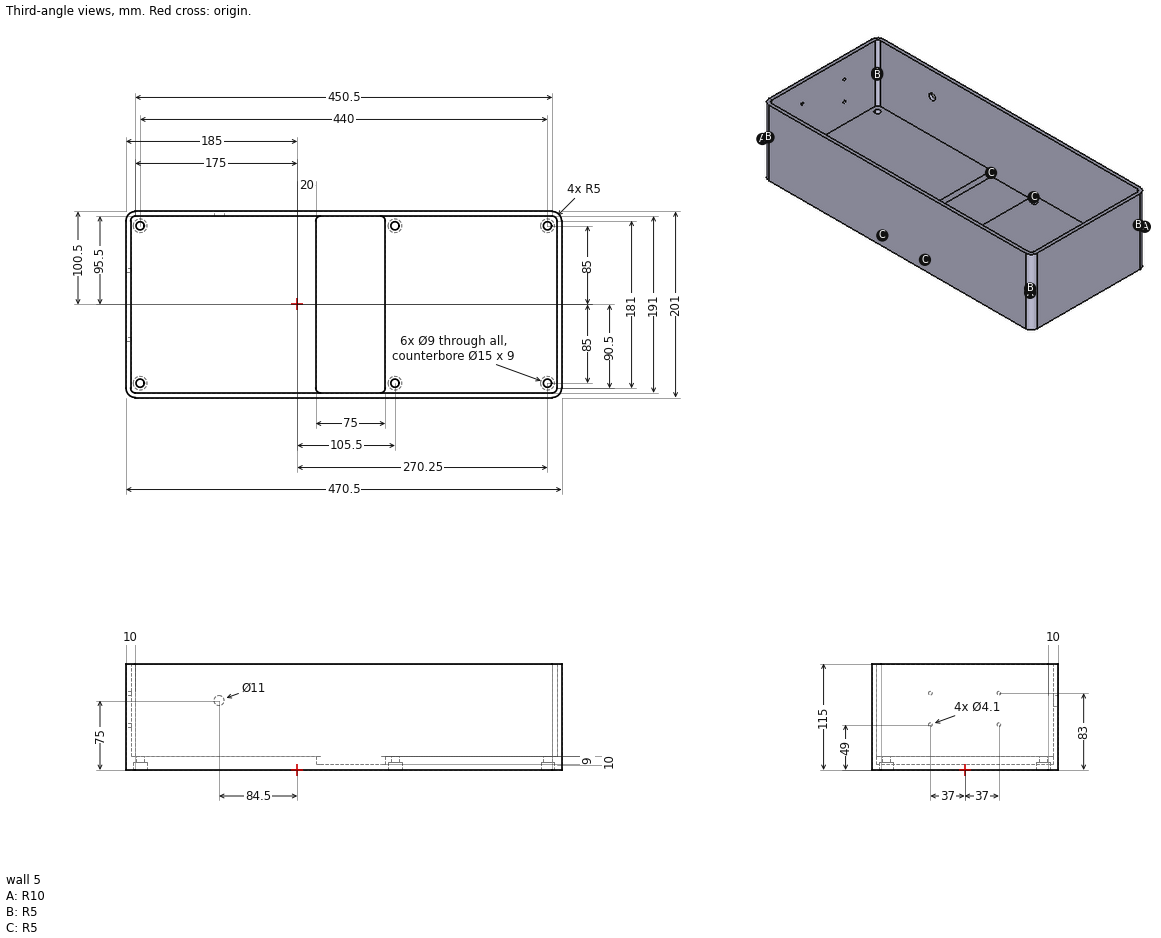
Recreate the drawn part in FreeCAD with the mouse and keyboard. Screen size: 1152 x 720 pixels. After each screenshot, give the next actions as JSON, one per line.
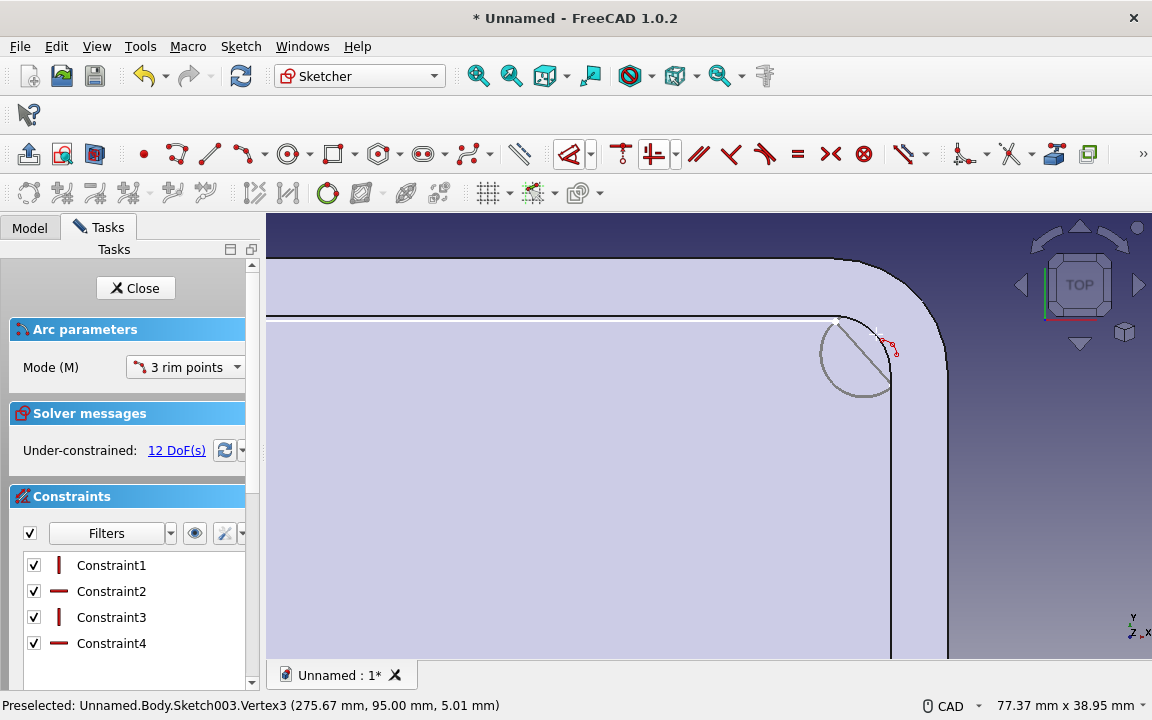
{"action": "left_click", "coordinate": [874, 332]}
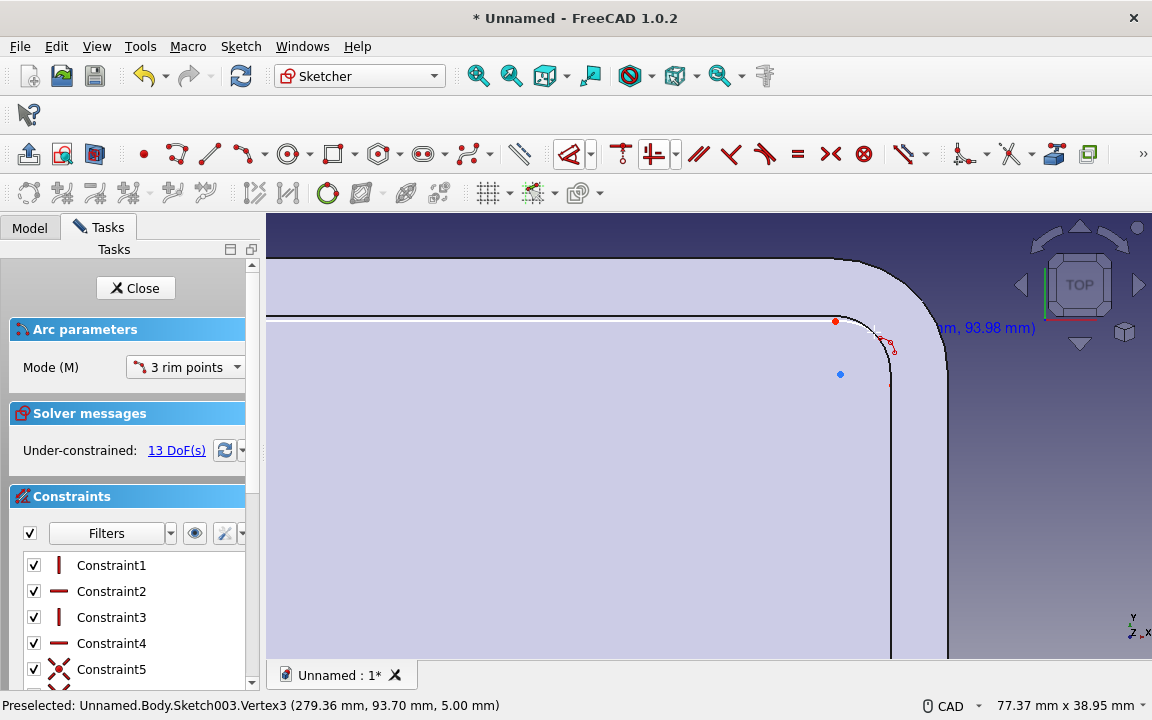
{"action": "scroll", "coordinate": [879, 339], "scroll_direction": "down", "scroll_amount": 12}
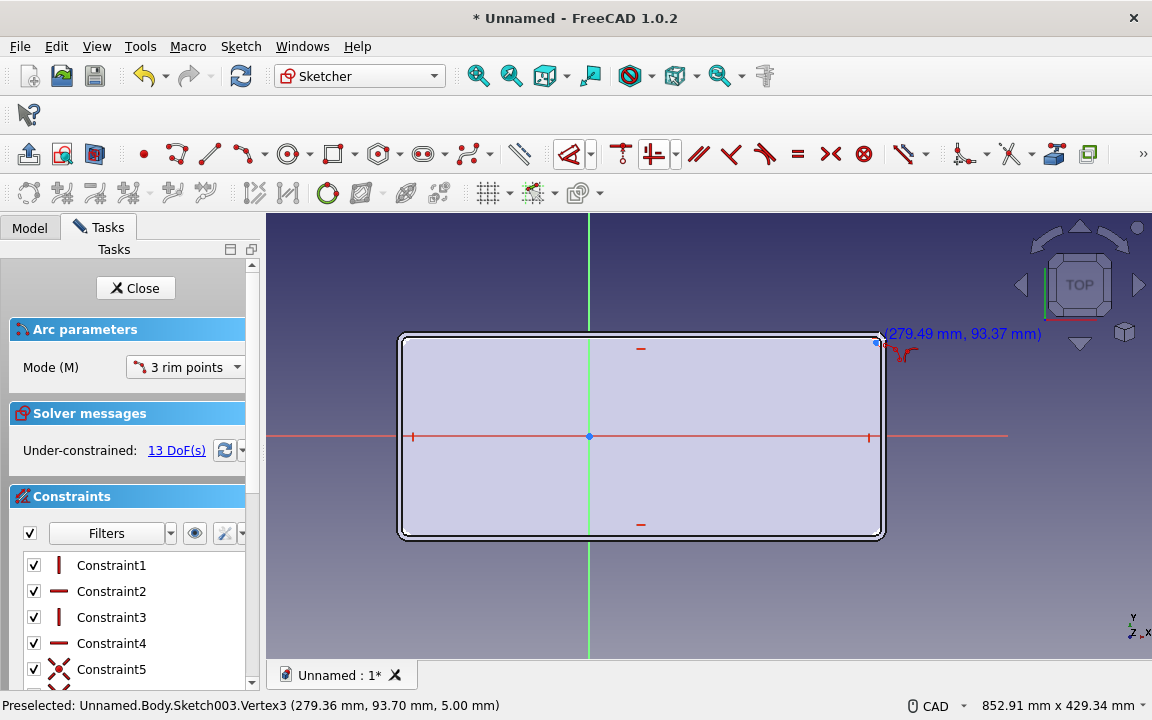
{"action": "scroll", "coordinate": [408, 337], "scroll_direction": "up", "scroll_amount": 4}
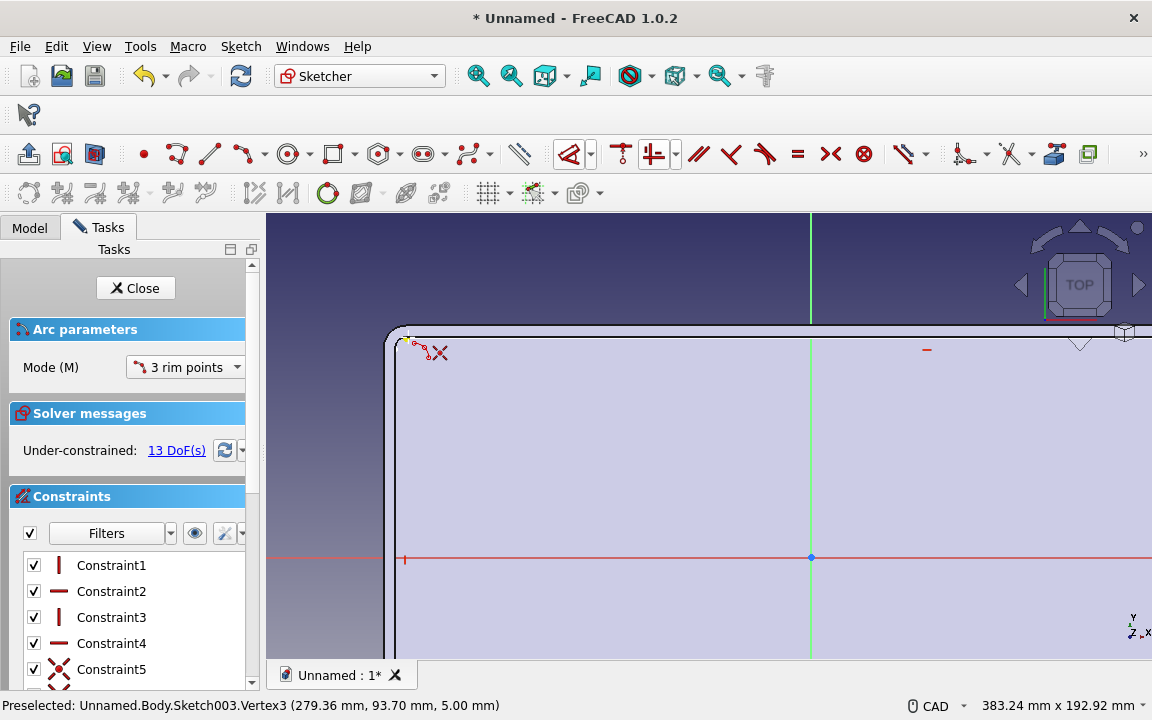
{"action": "left_click", "coordinate": [407, 338]}
{"action": "left_click", "coordinate": [395, 349]}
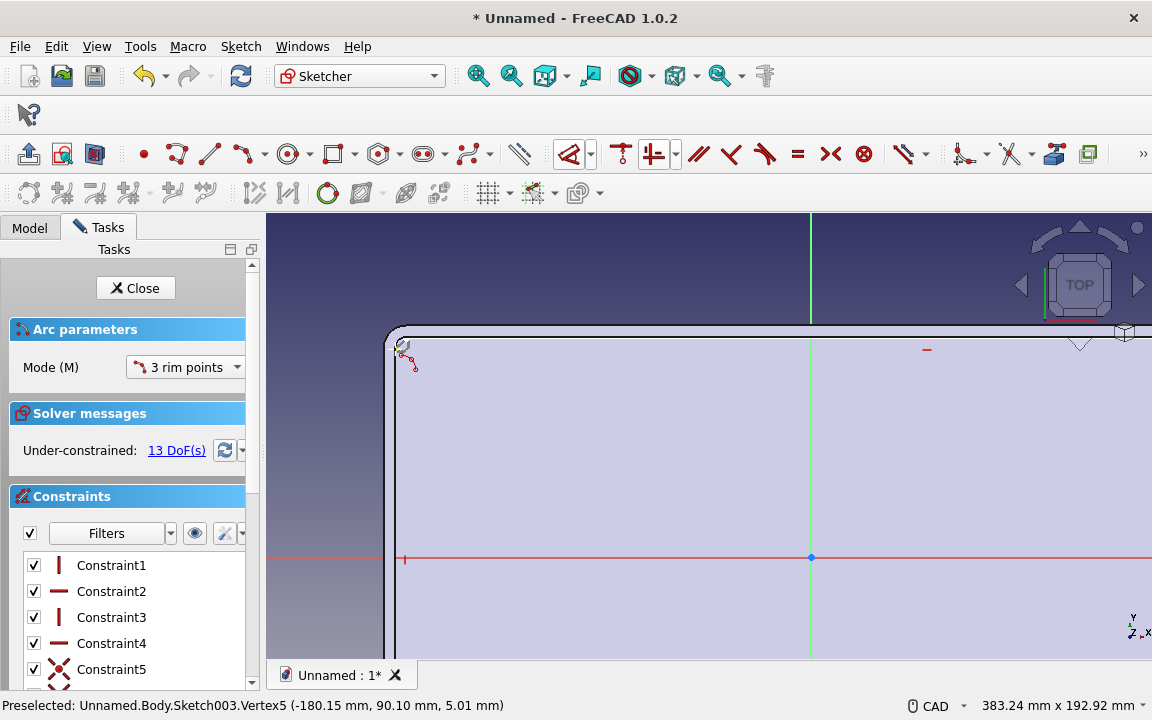
{"action": "scroll", "coordinate": [399, 340], "scroll_direction": "up", "scroll_amount": 8}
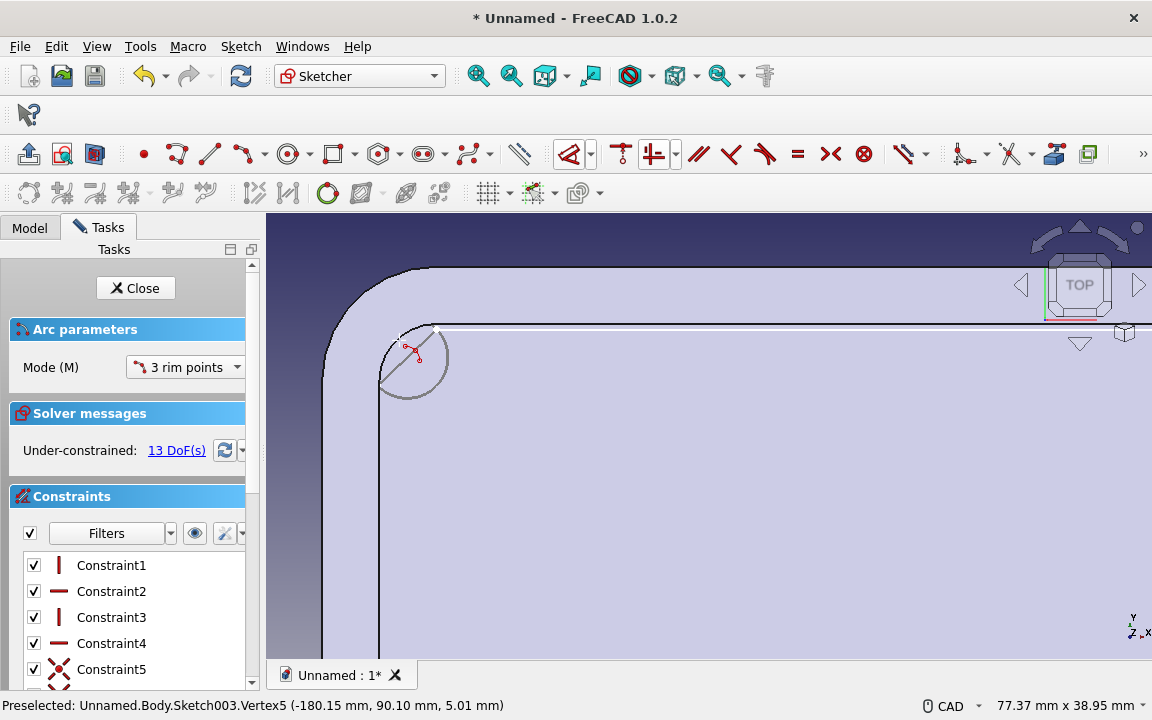
{"action": "left_click", "coordinate": [396, 341]}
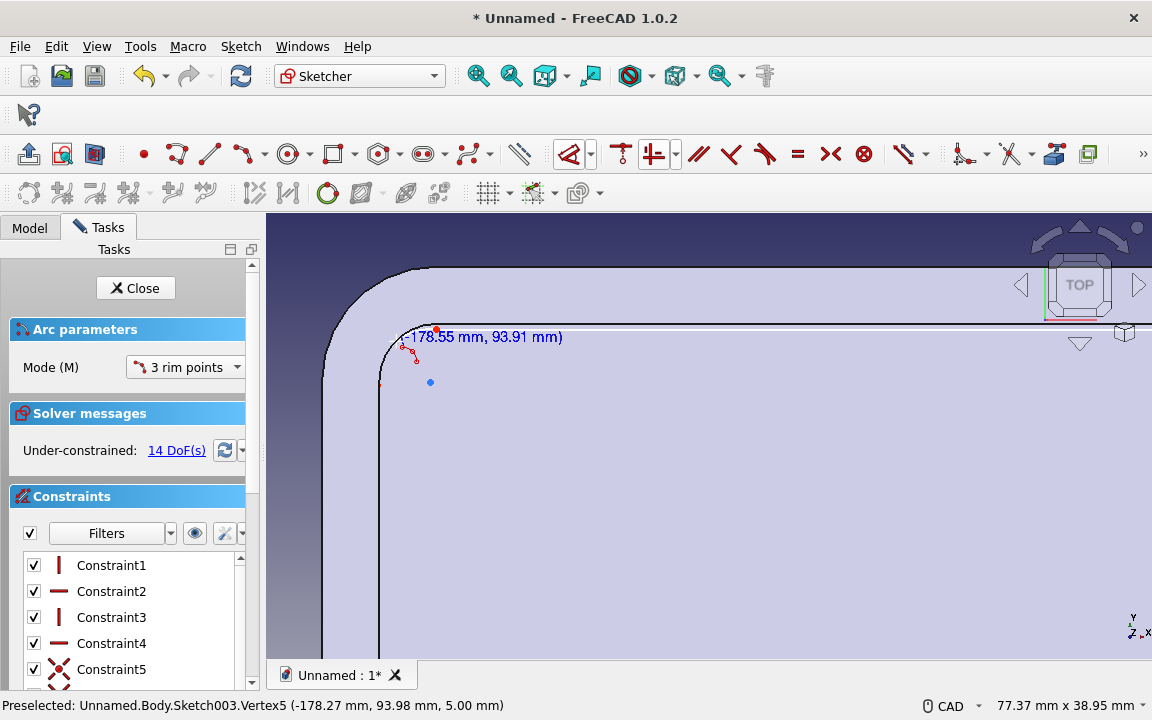
{"action": "scroll", "coordinate": [404, 338], "scroll_direction": "down", "scroll_amount": 12}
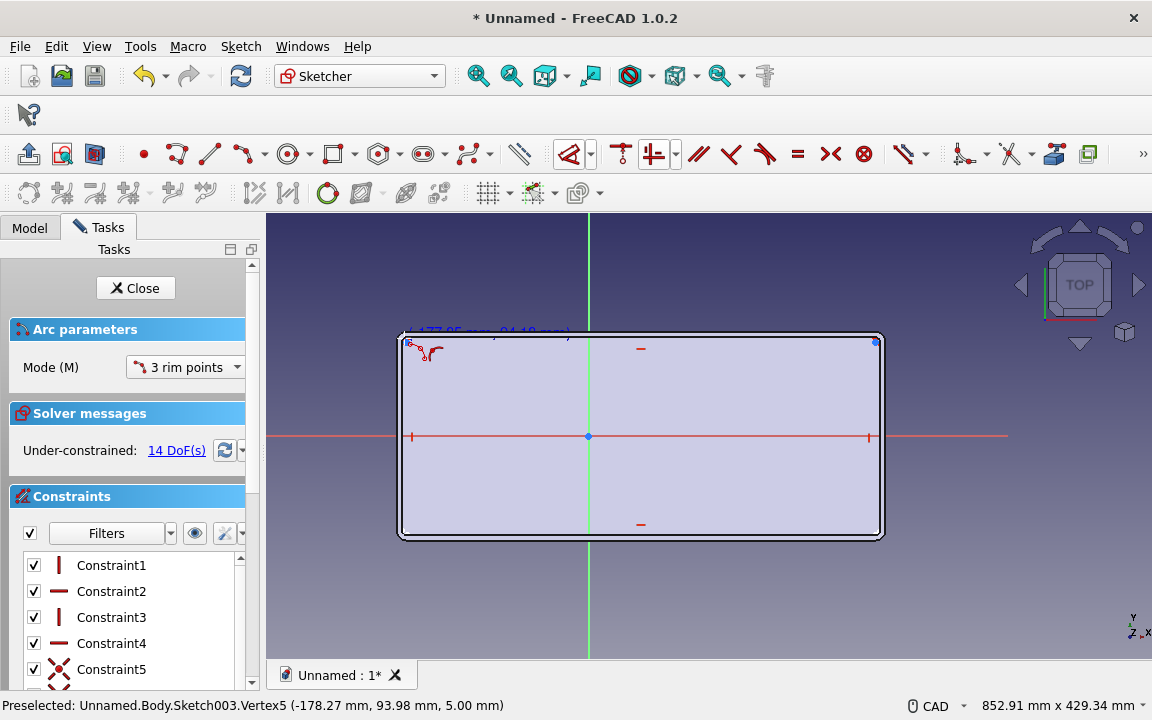
{"action": "scroll", "coordinate": [402, 530], "scroll_direction": "up", "scroll_amount": 4}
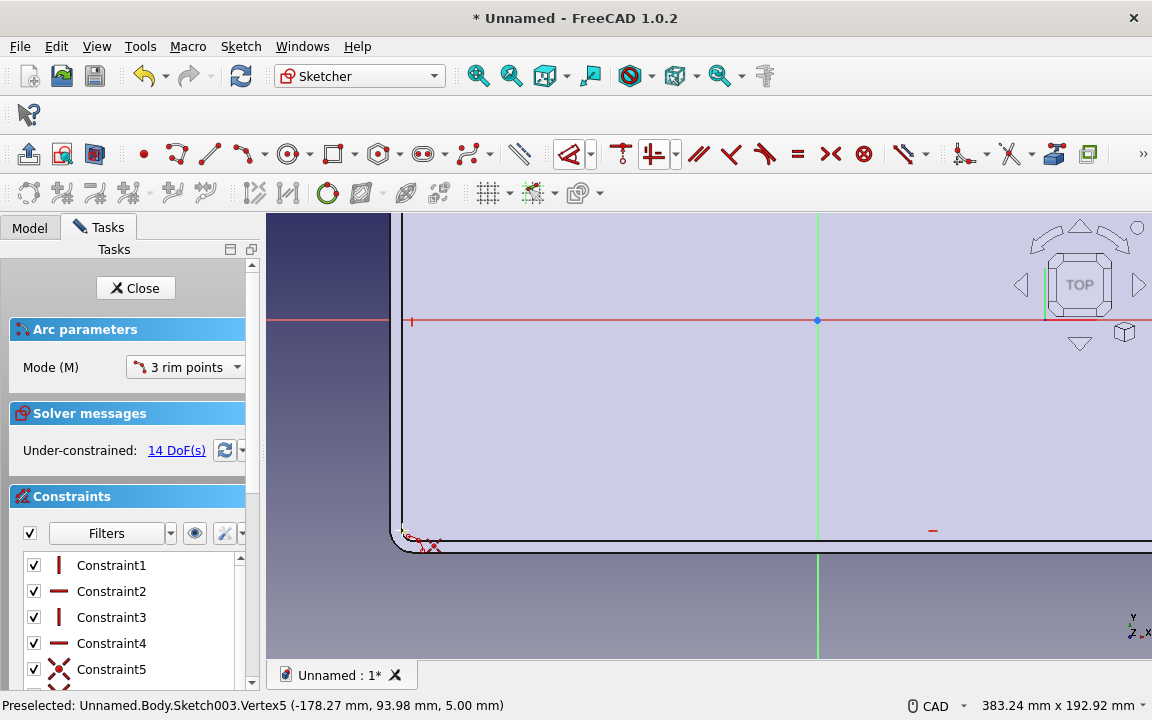
{"action": "left_click", "coordinate": [401, 531]}
{"action": "left_click", "coordinate": [413, 542]}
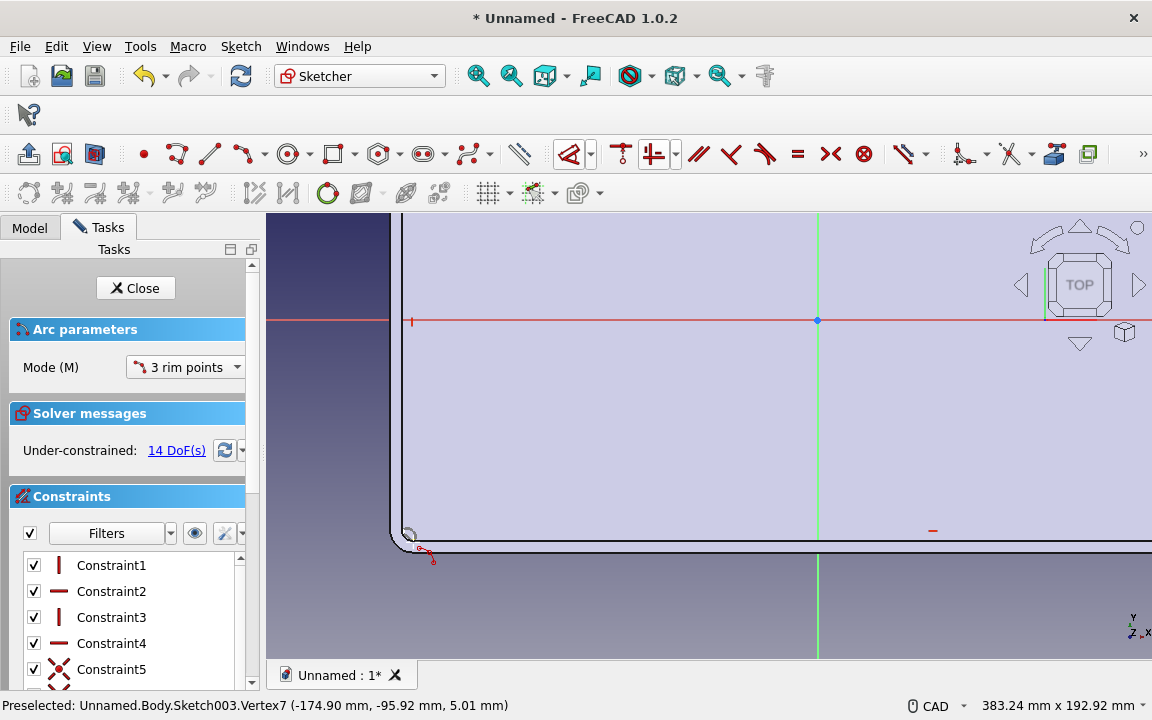
{"action": "scroll", "coordinate": [405, 538], "scroll_direction": "up", "scroll_amount": 8}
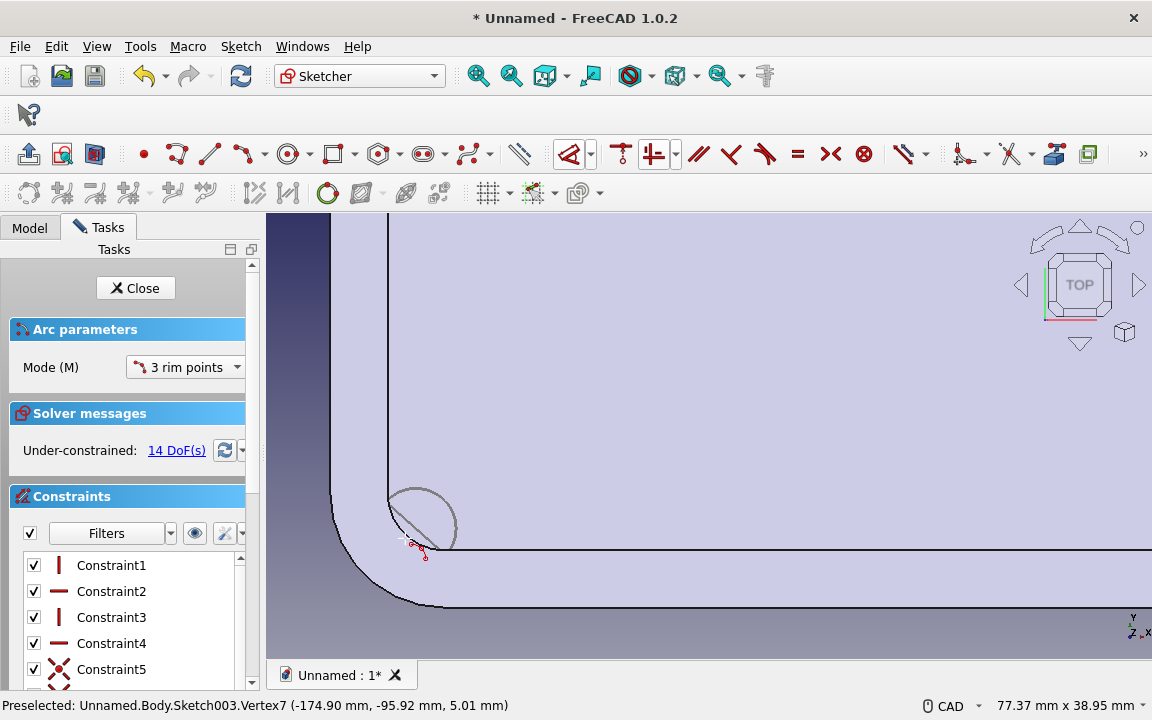
{"action": "left_click", "coordinate": [404, 534]}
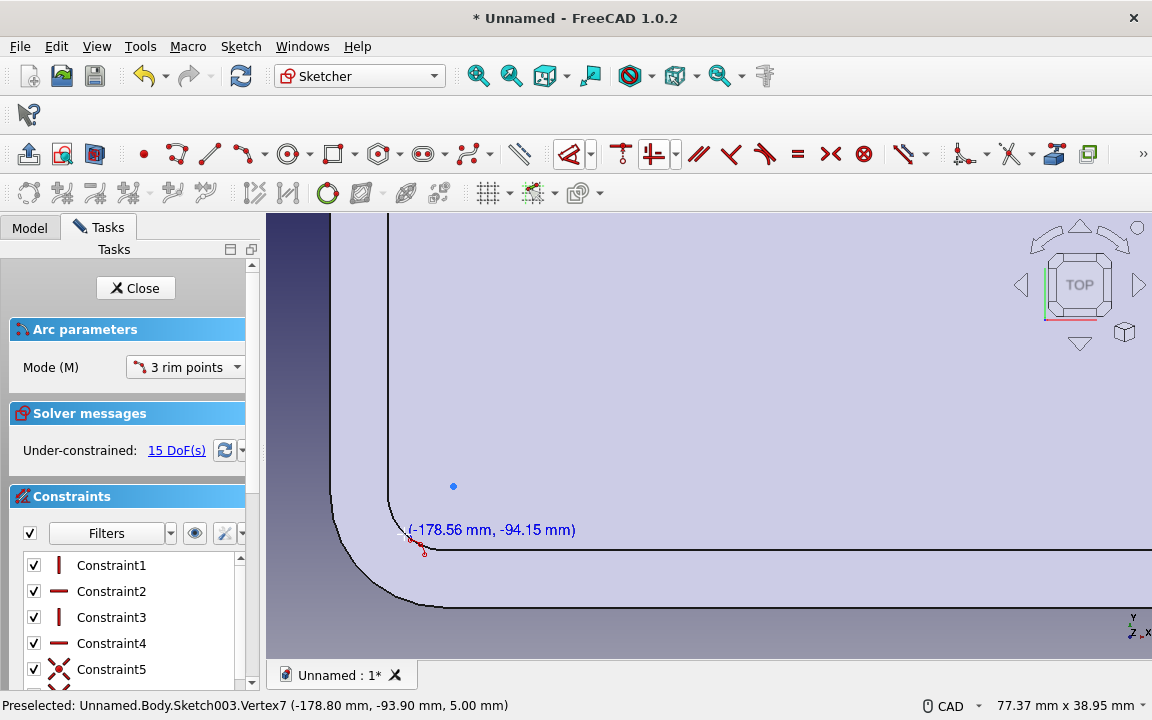
{"action": "scroll", "coordinate": [403, 534], "scroll_direction": "down", "scroll_amount": 12}